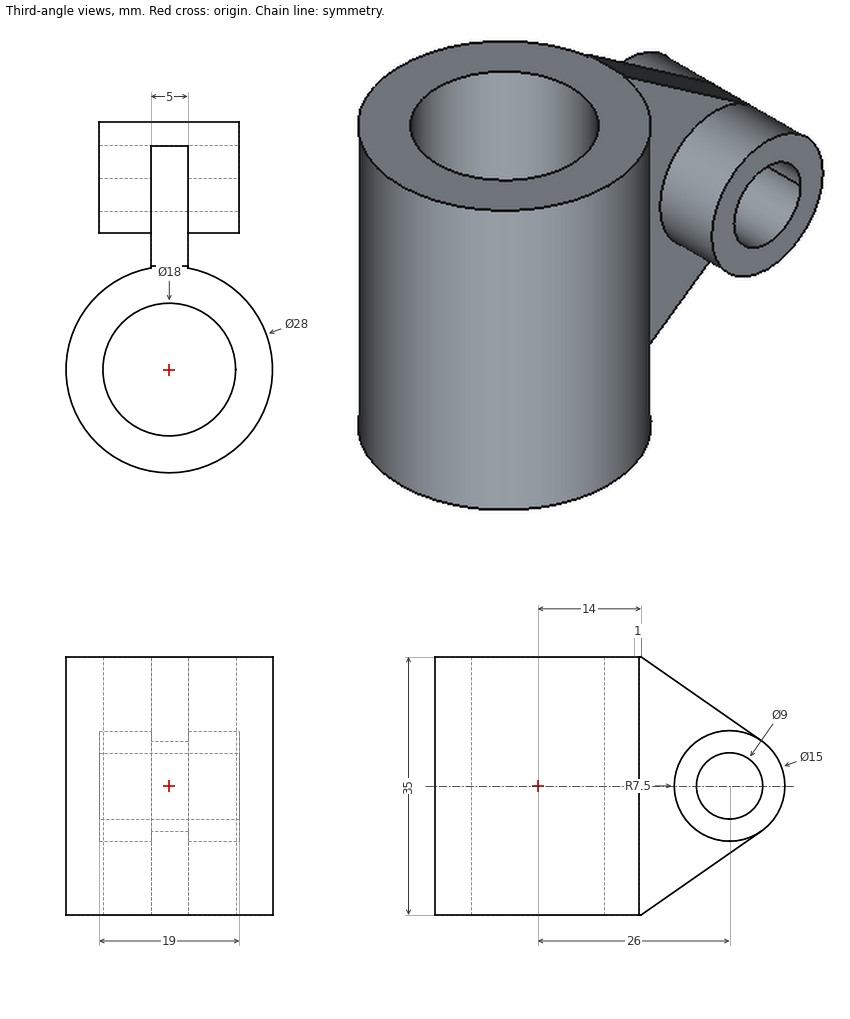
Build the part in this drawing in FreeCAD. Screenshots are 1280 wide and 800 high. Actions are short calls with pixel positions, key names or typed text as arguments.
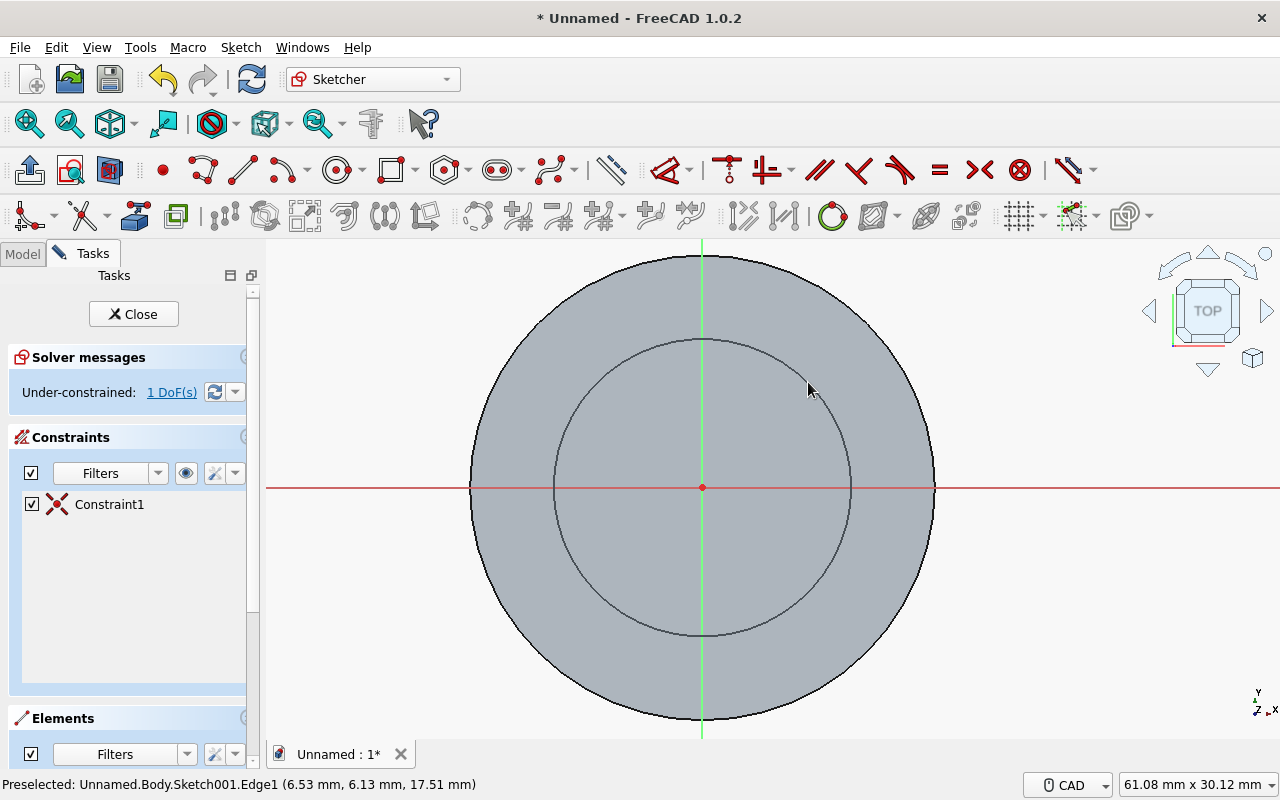
click(666, 170)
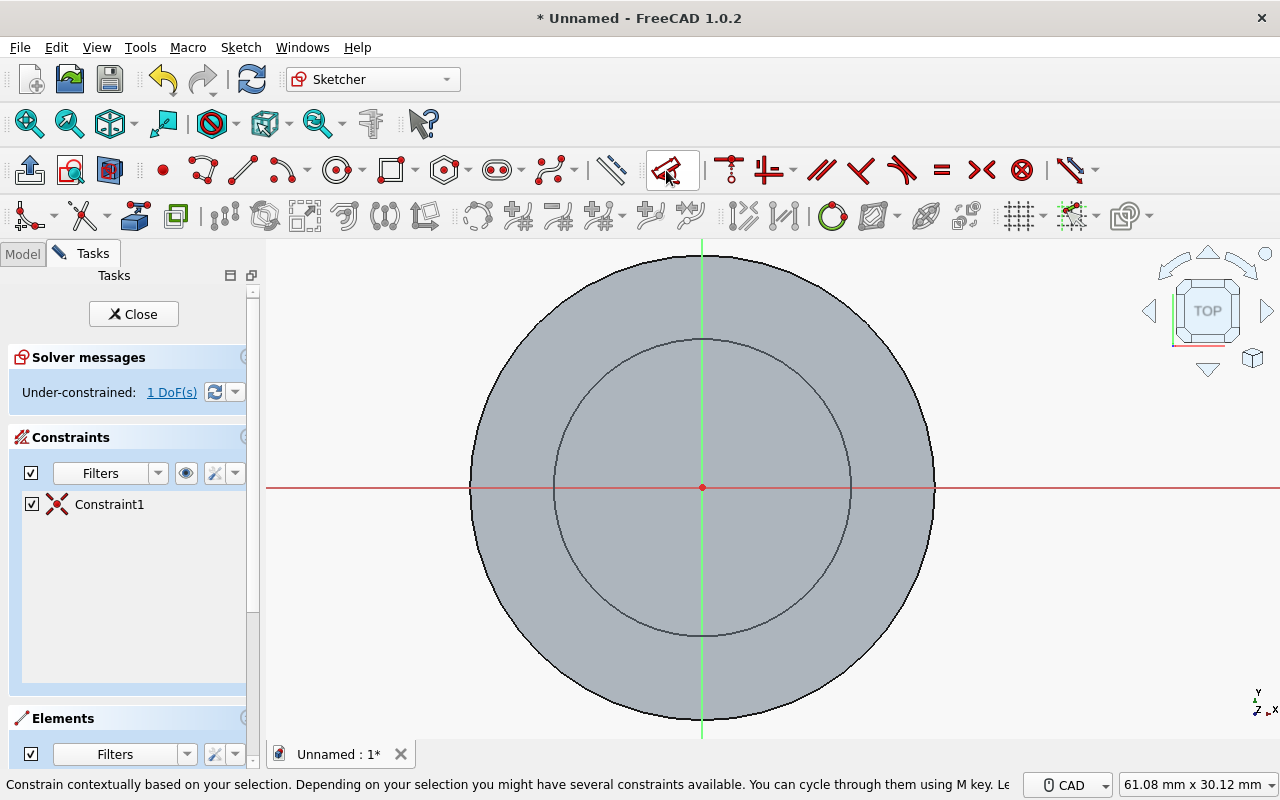
click(807, 382)
click(829, 359)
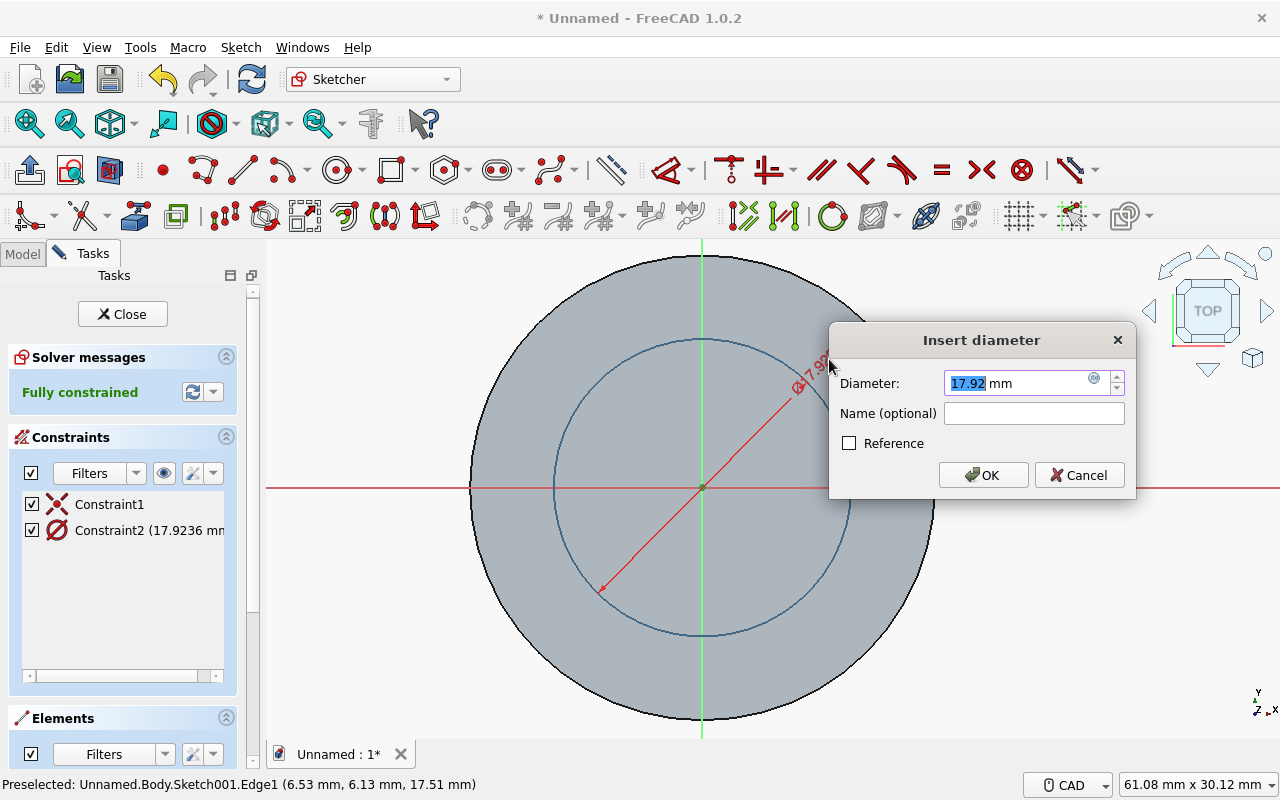
text(18)
key(Return)
key(Escape)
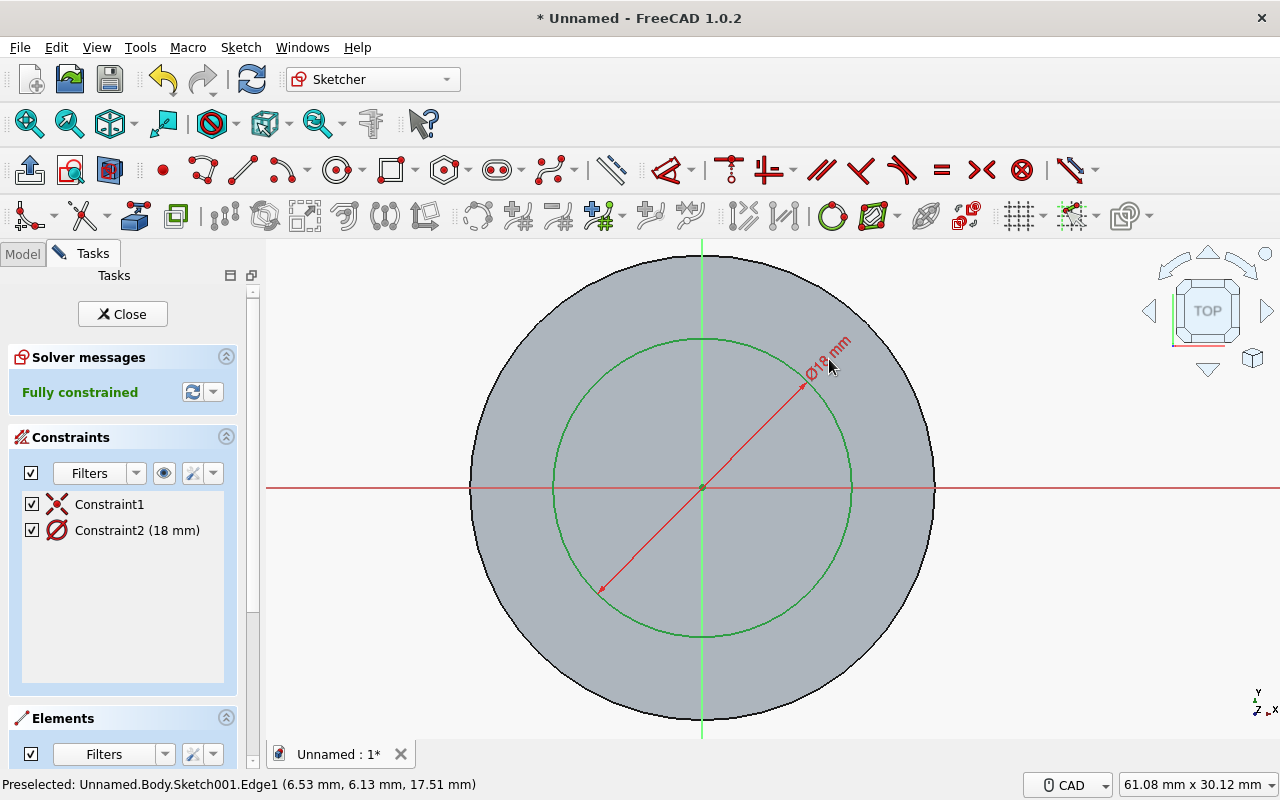
click(123, 314)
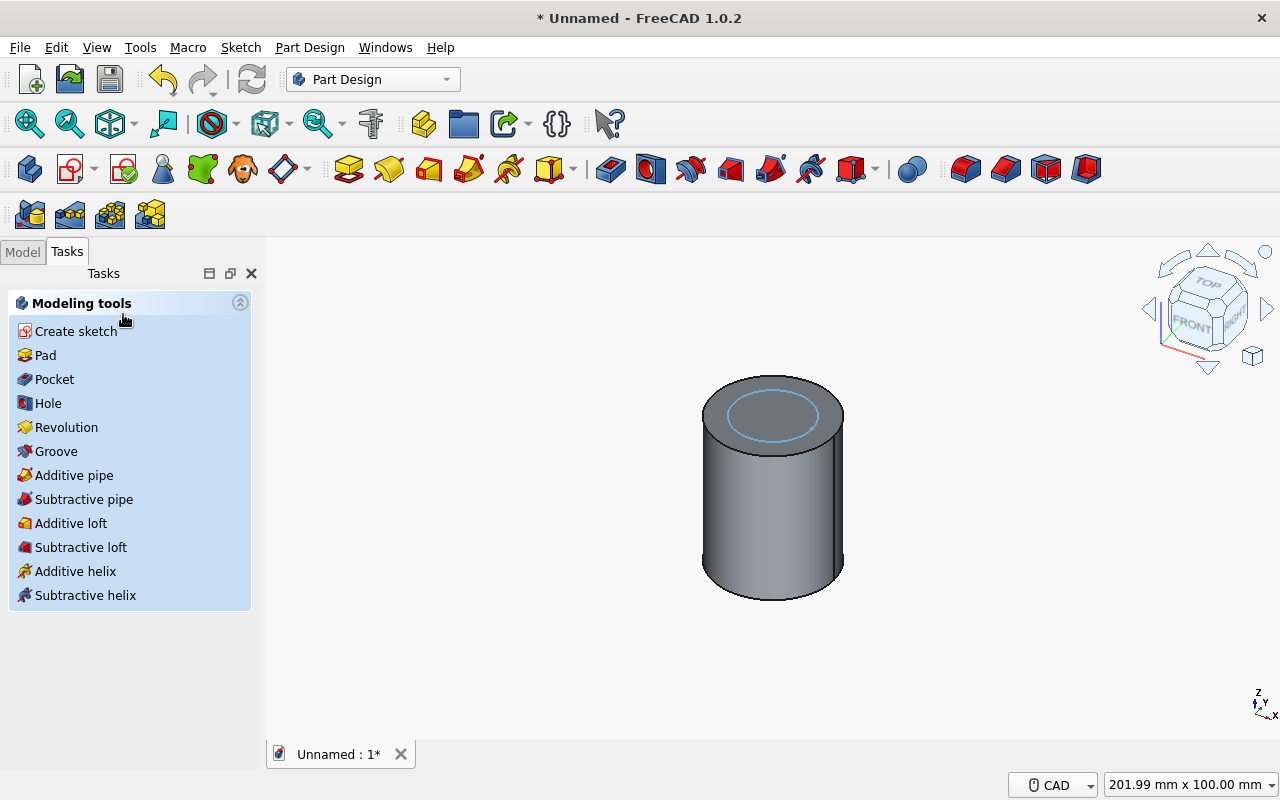
click(612, 170)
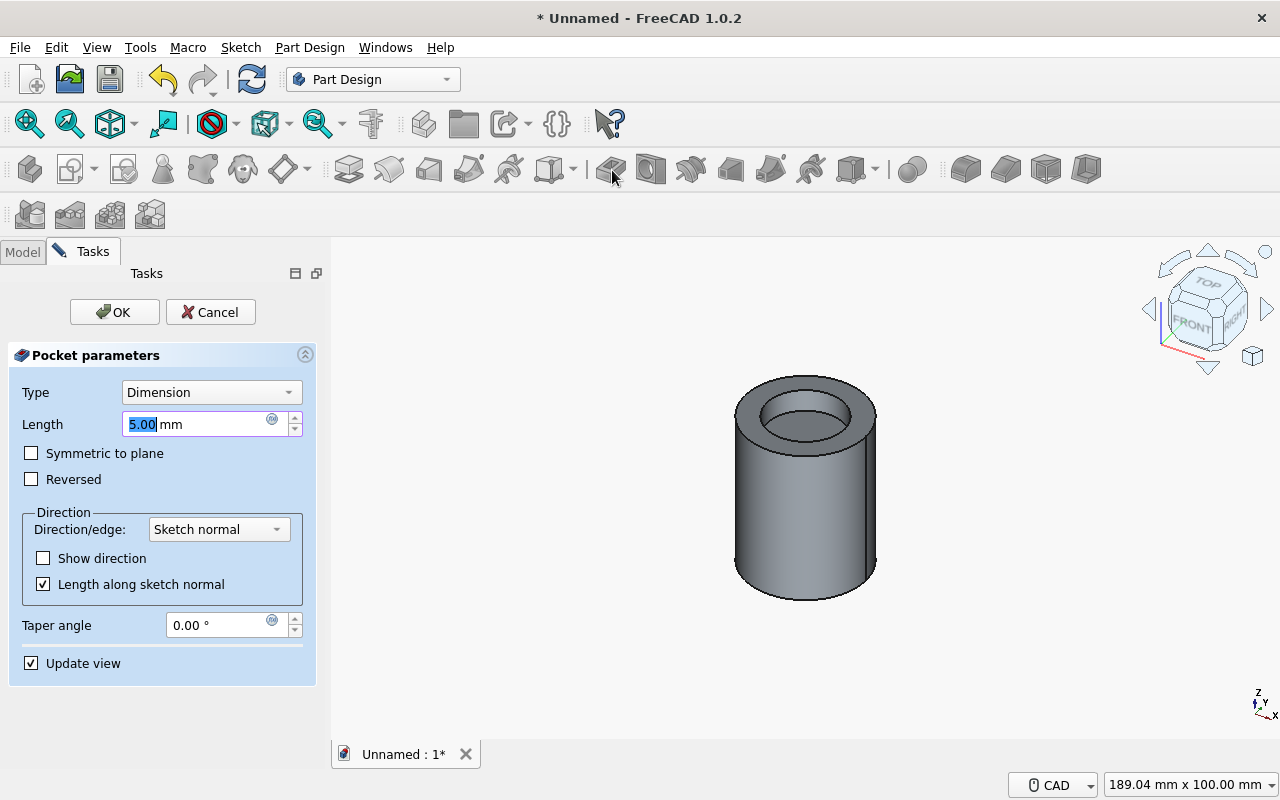
click(212, 392)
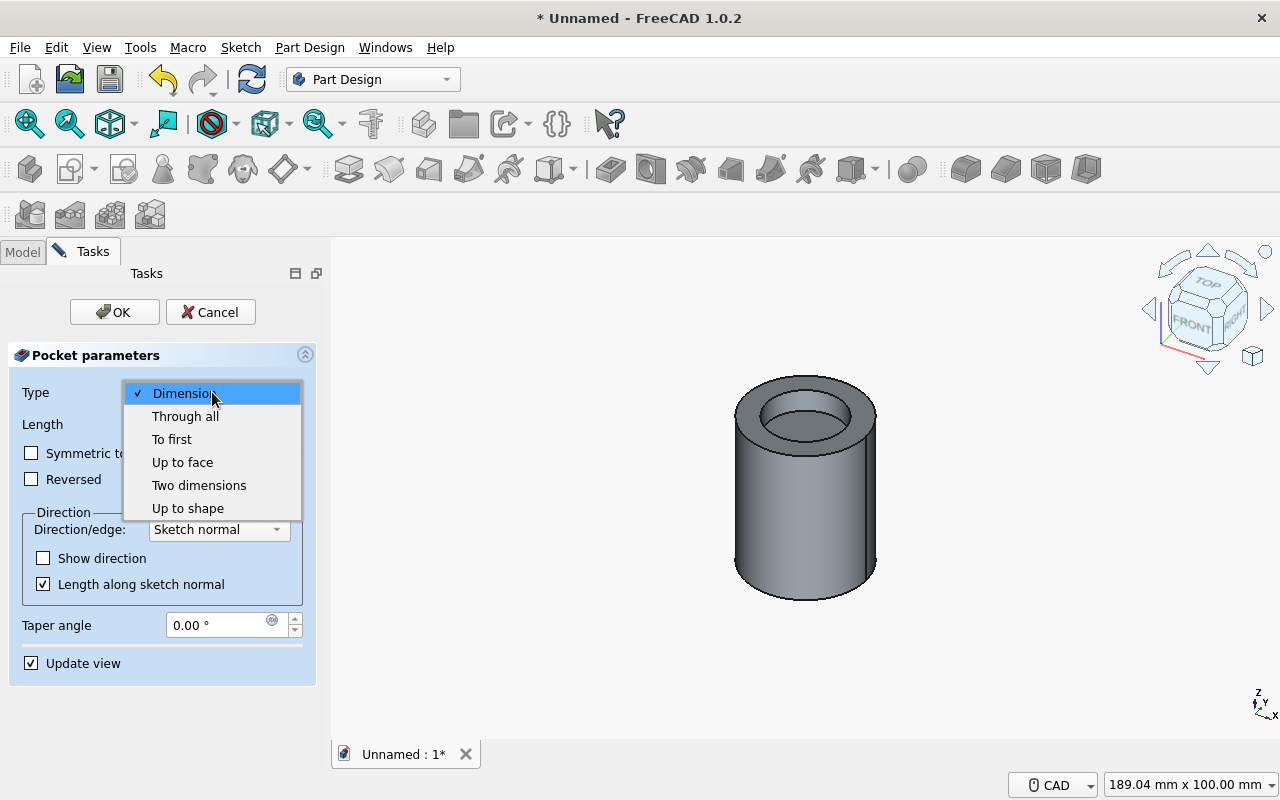
click(212, 416)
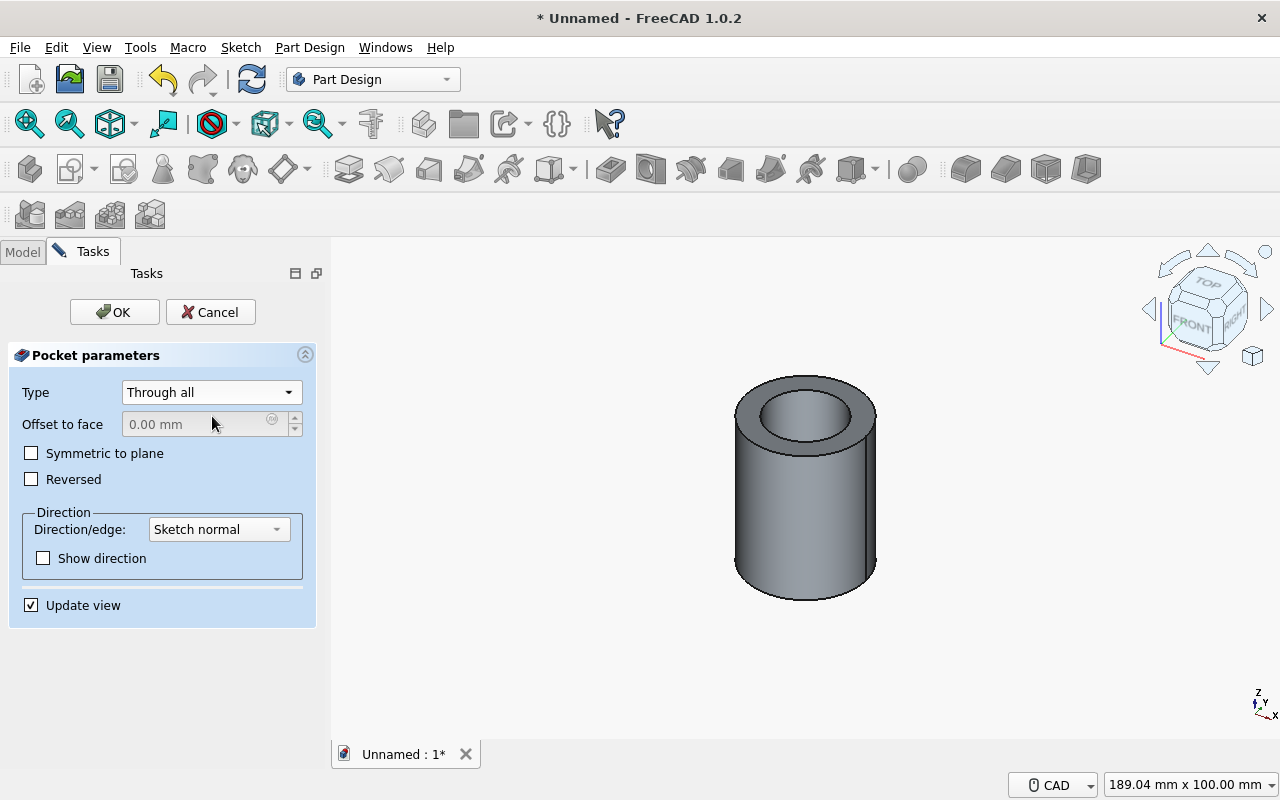
click(115, 312)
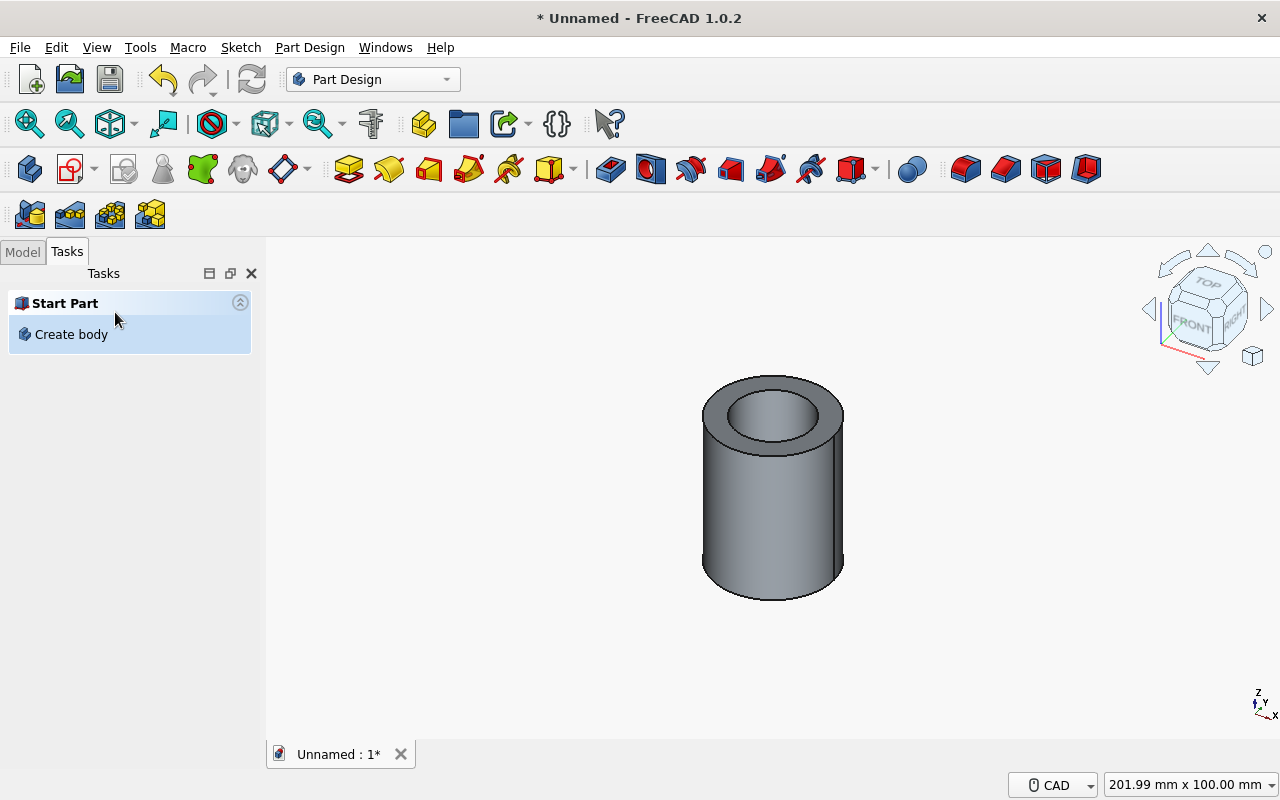
click(30, 170)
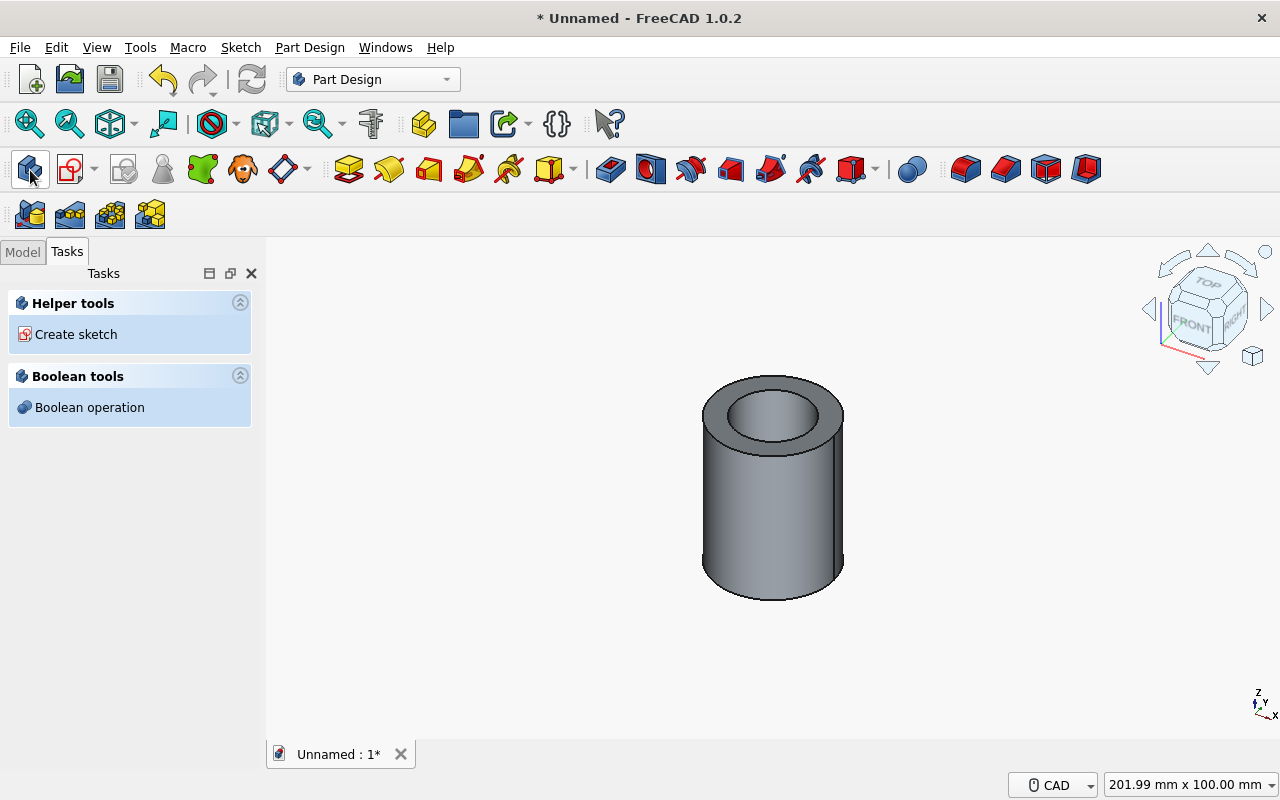
click(306, 699)